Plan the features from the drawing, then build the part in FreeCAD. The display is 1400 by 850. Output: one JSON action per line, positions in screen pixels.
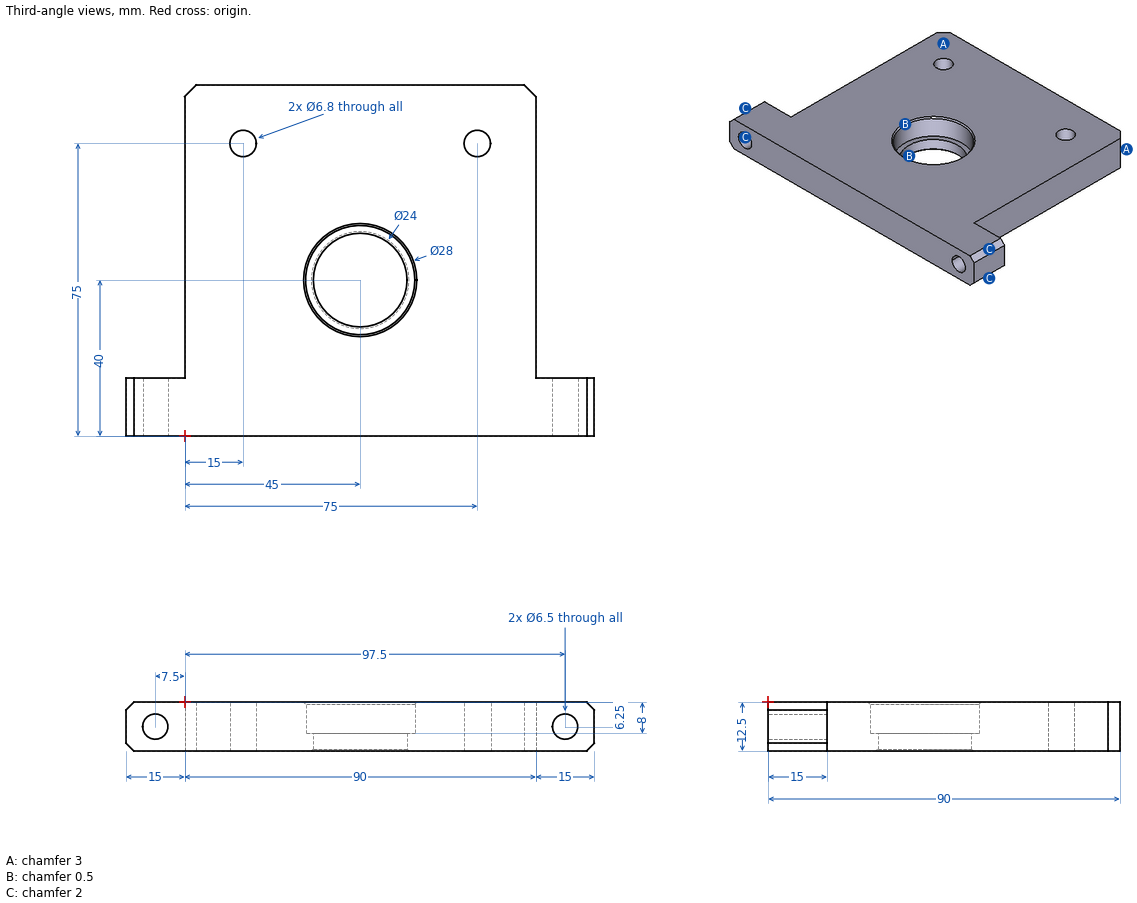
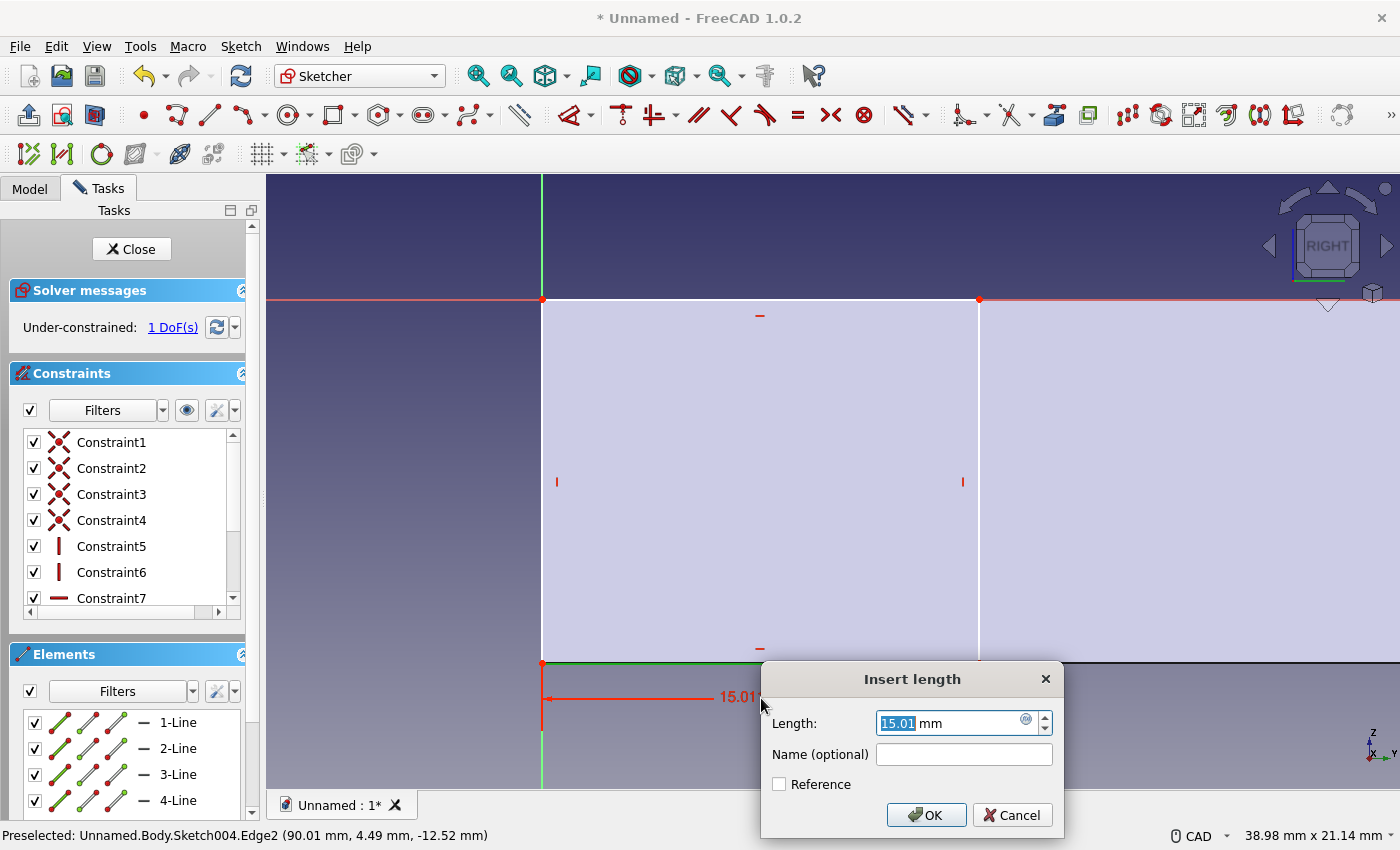
{"action": "type", "text": "15"}
{"action": "key", "text": "Return"}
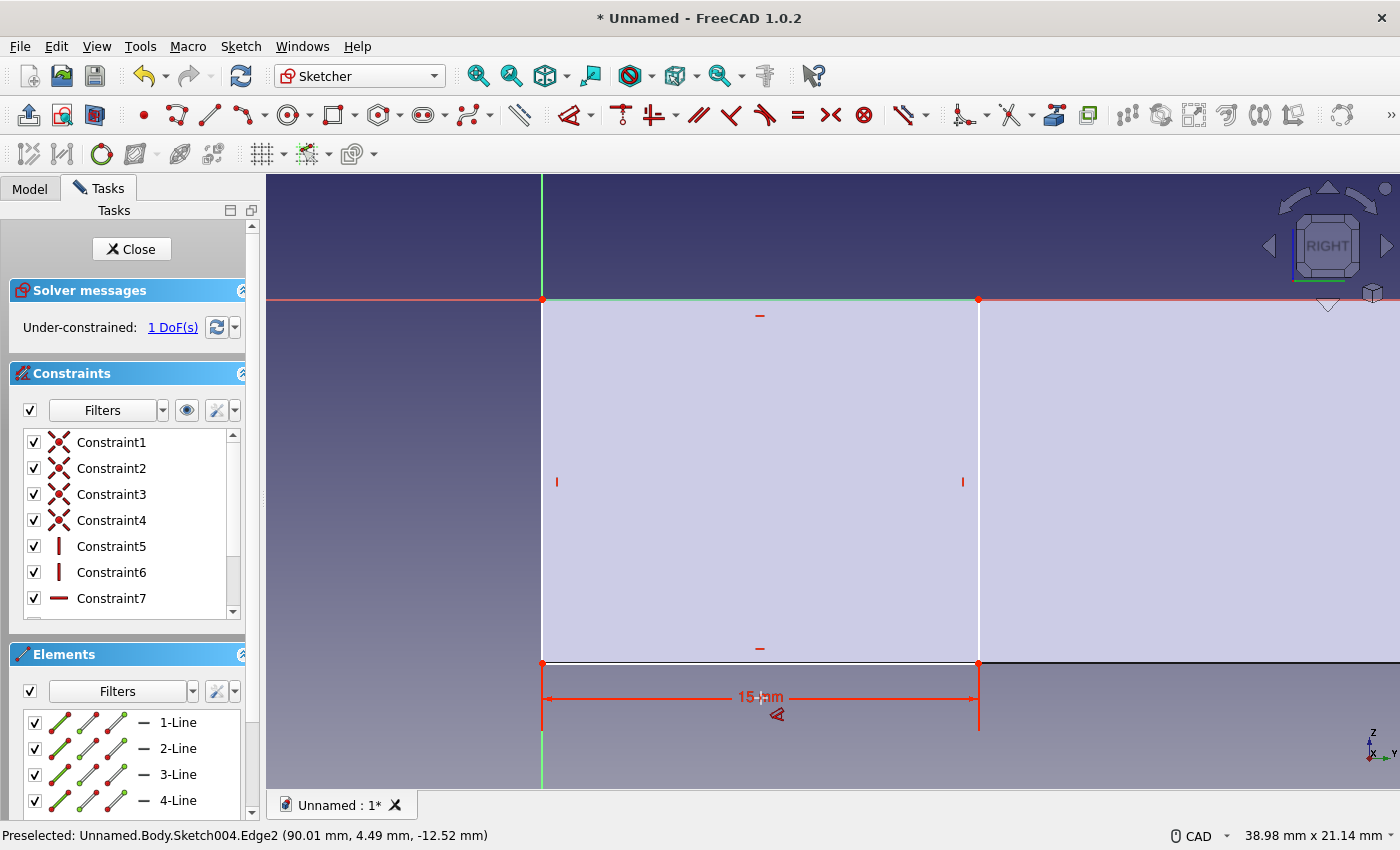
{"action": "left_click", "coordinate": [542, 409]}
{"action": "left_click", "coordinate": [508, 482]}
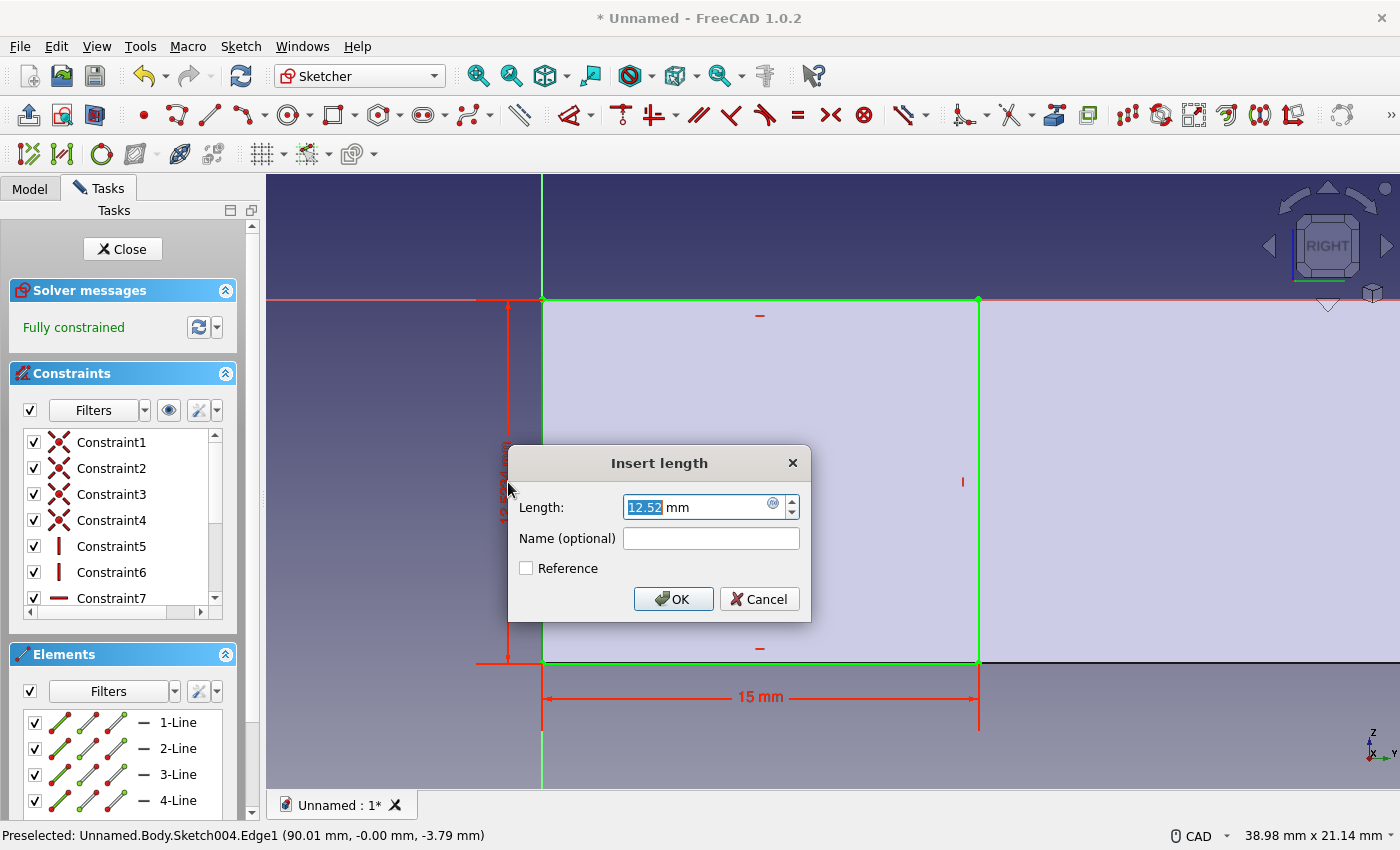
{"action": "type", "text": "12.5"}
{"action": "key", "text": "Return"}
{"action": "key", "text": "Escape"}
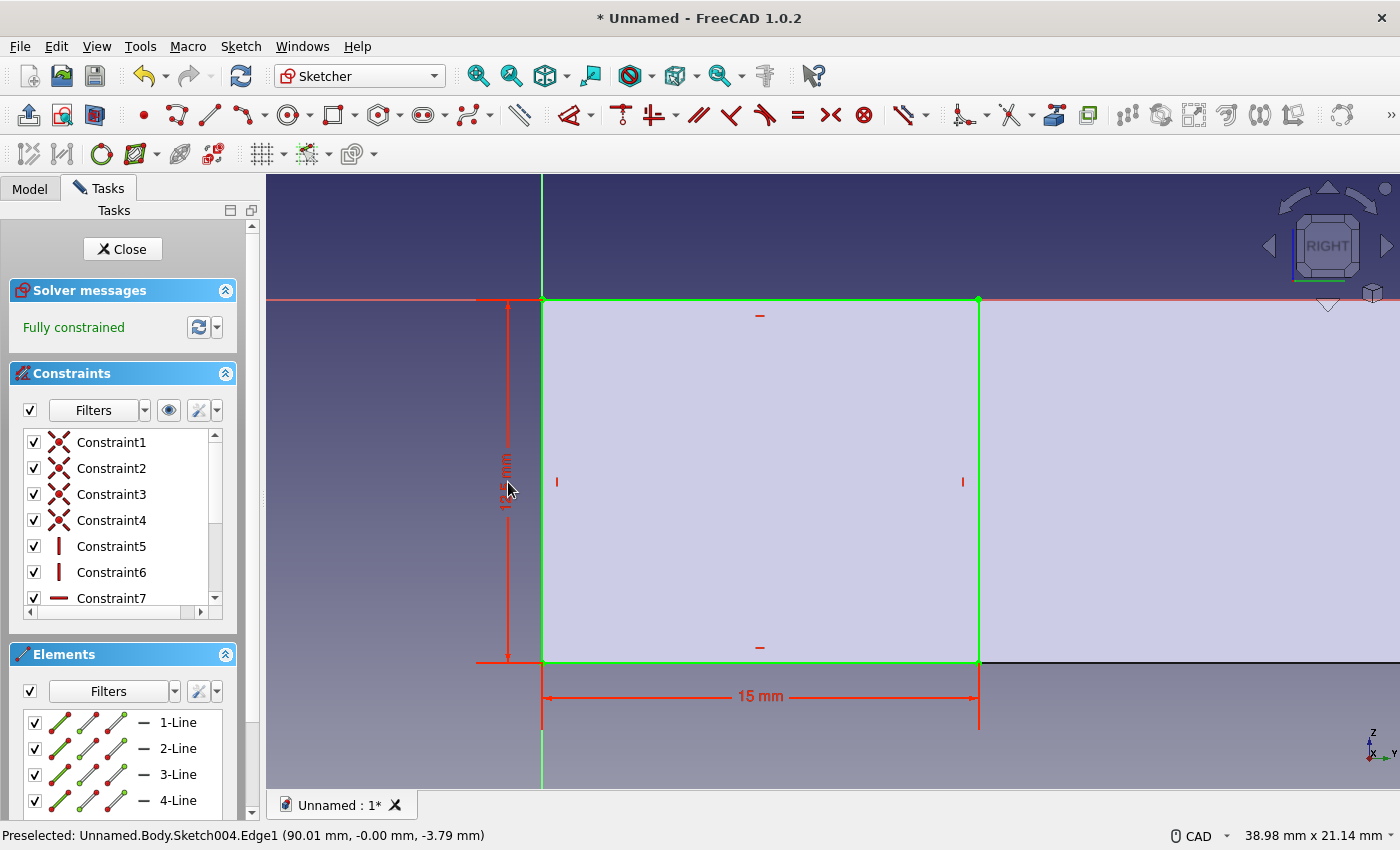
{"action": "left_click", "coordinate": [123, 249]}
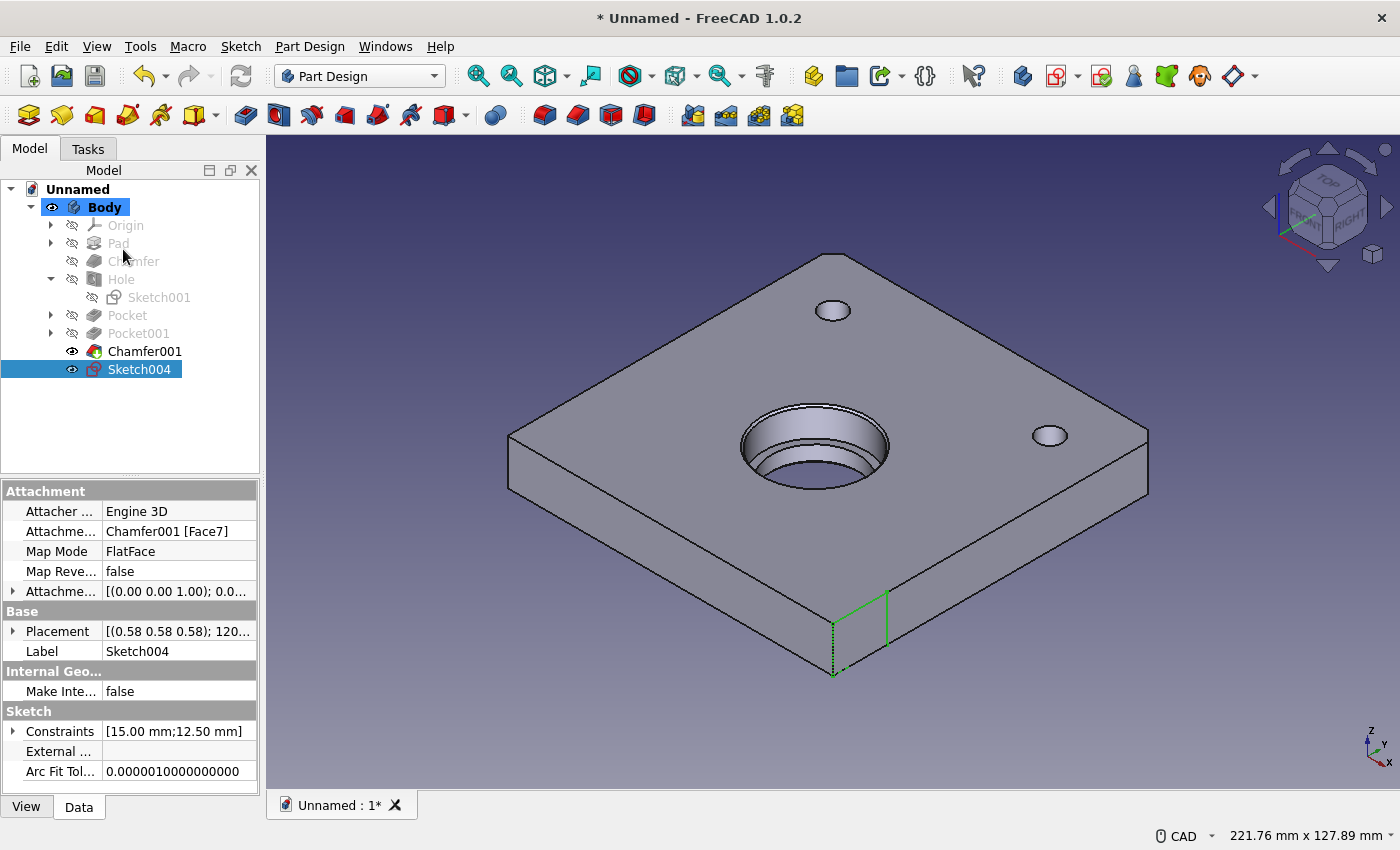
{"action": "left_click", "coordinate": [29, 116]}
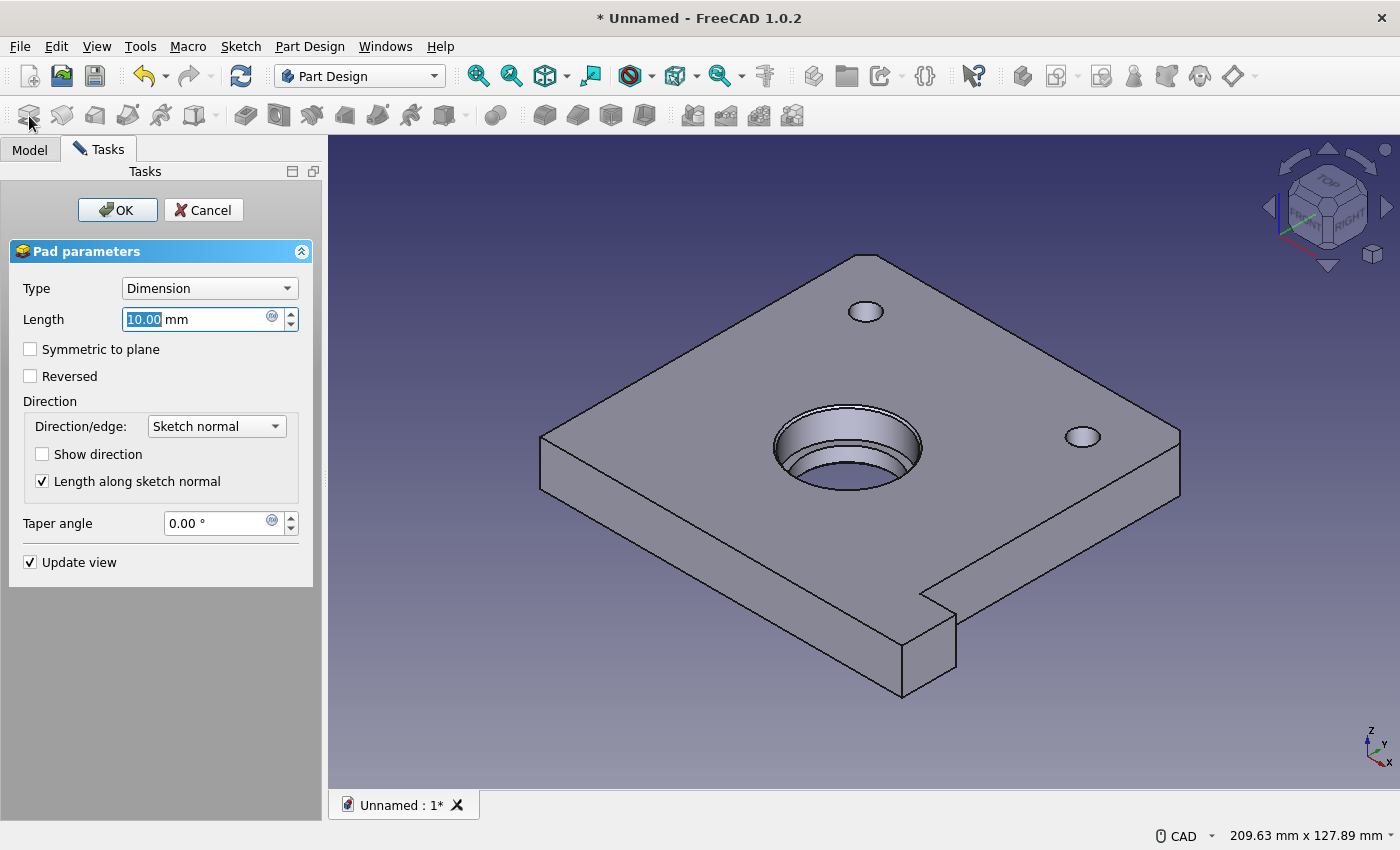
{"action": "type", "text": "15"}
{"action": "key", "text": "Tab"}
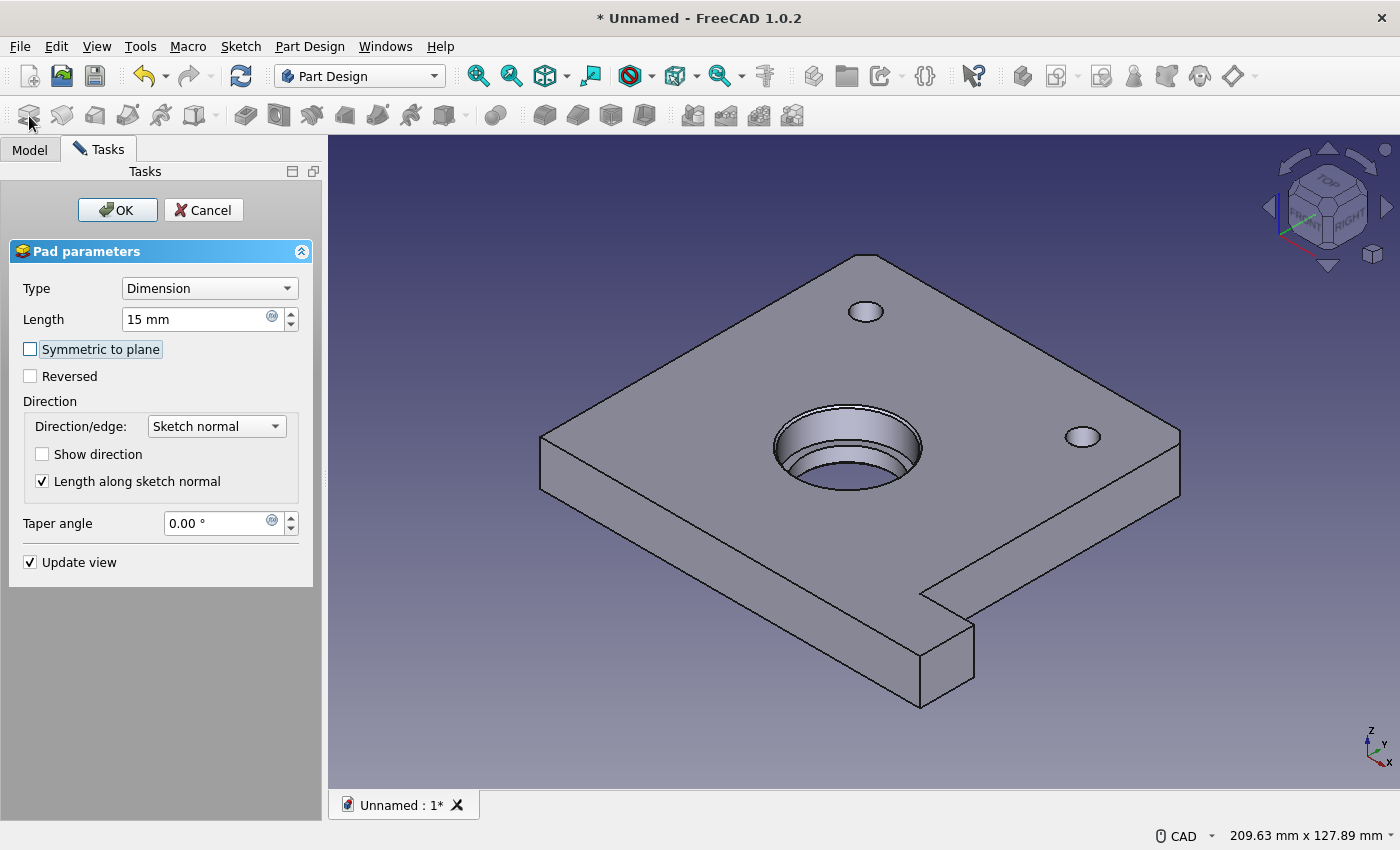
{"action": "left_click", "coordinate": [118, 210]}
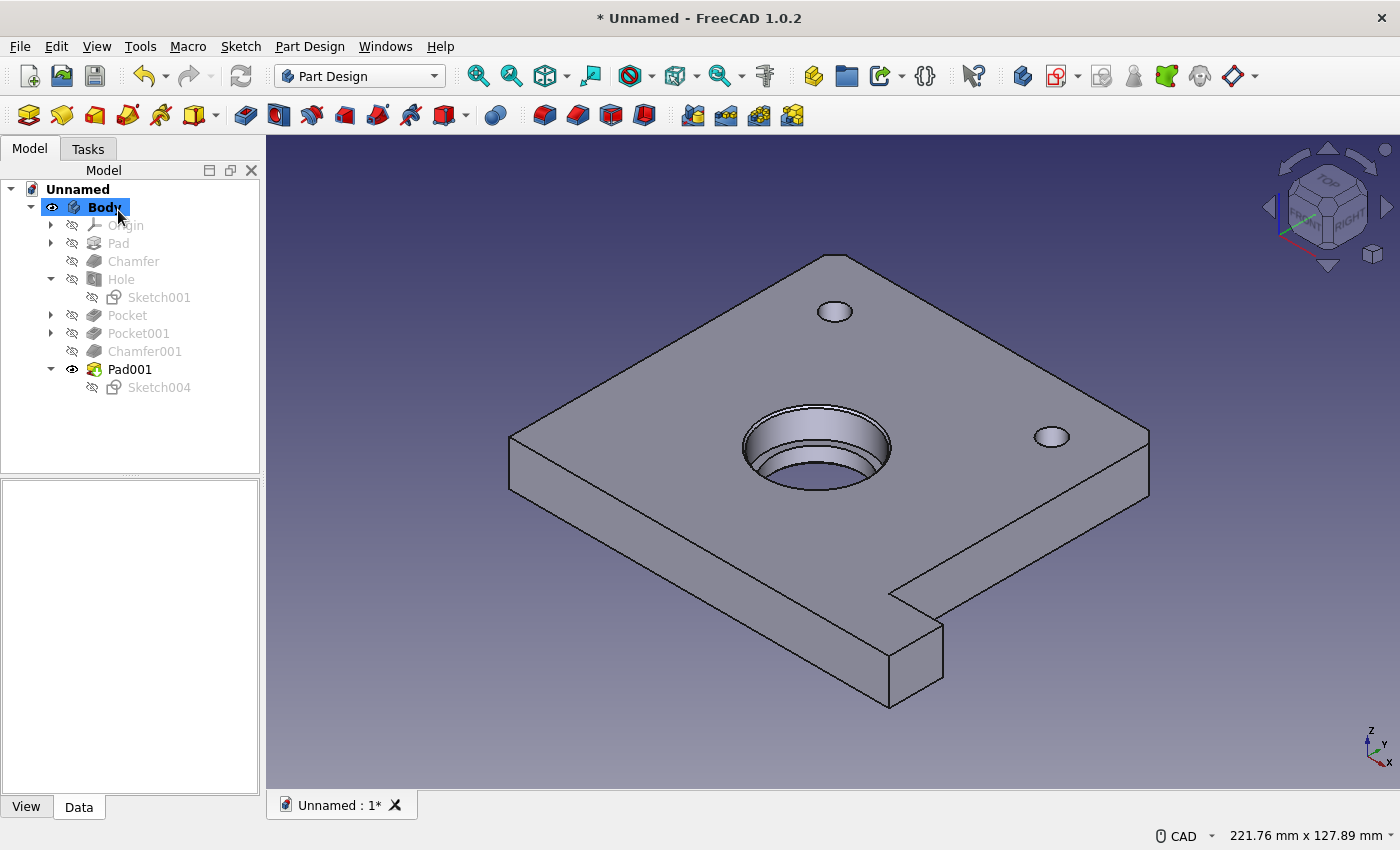
{"action": "key", "text": "6"}